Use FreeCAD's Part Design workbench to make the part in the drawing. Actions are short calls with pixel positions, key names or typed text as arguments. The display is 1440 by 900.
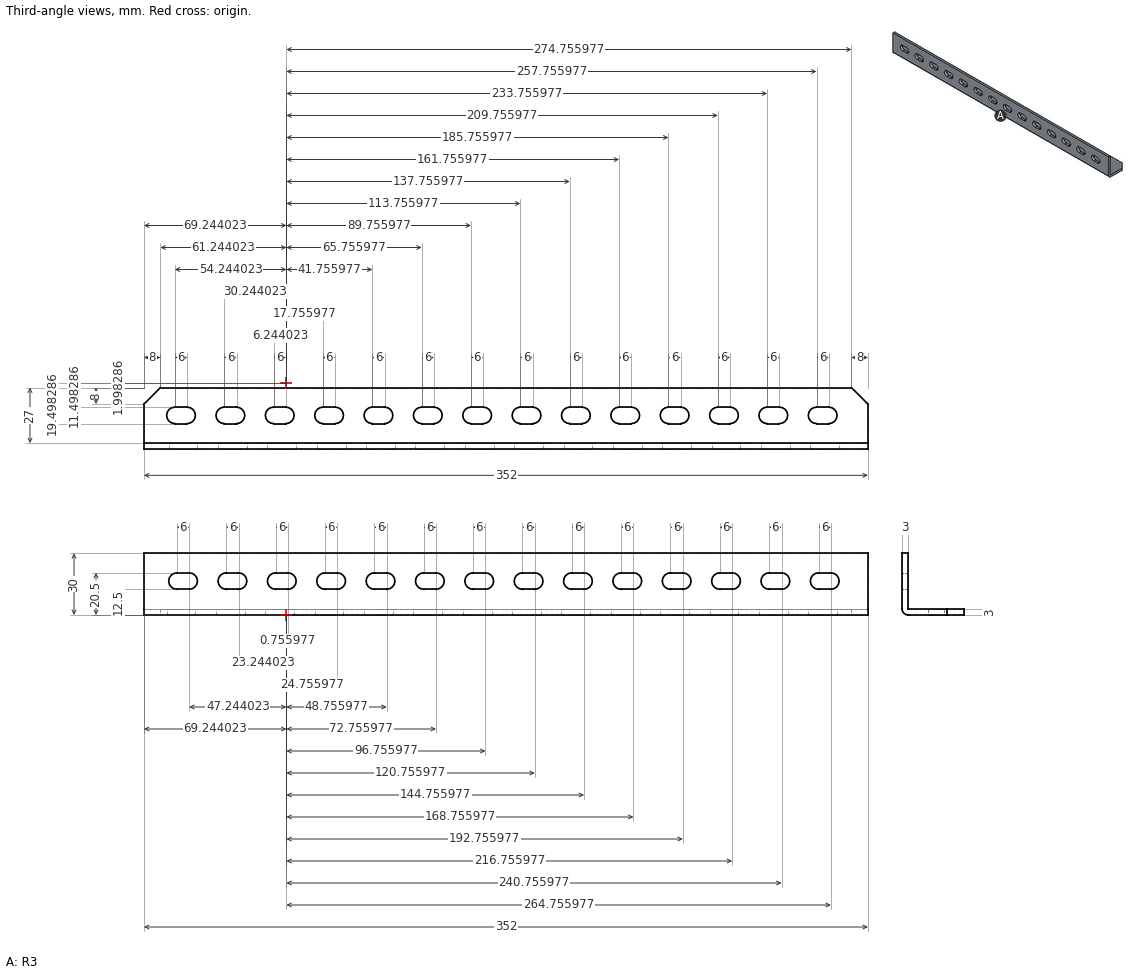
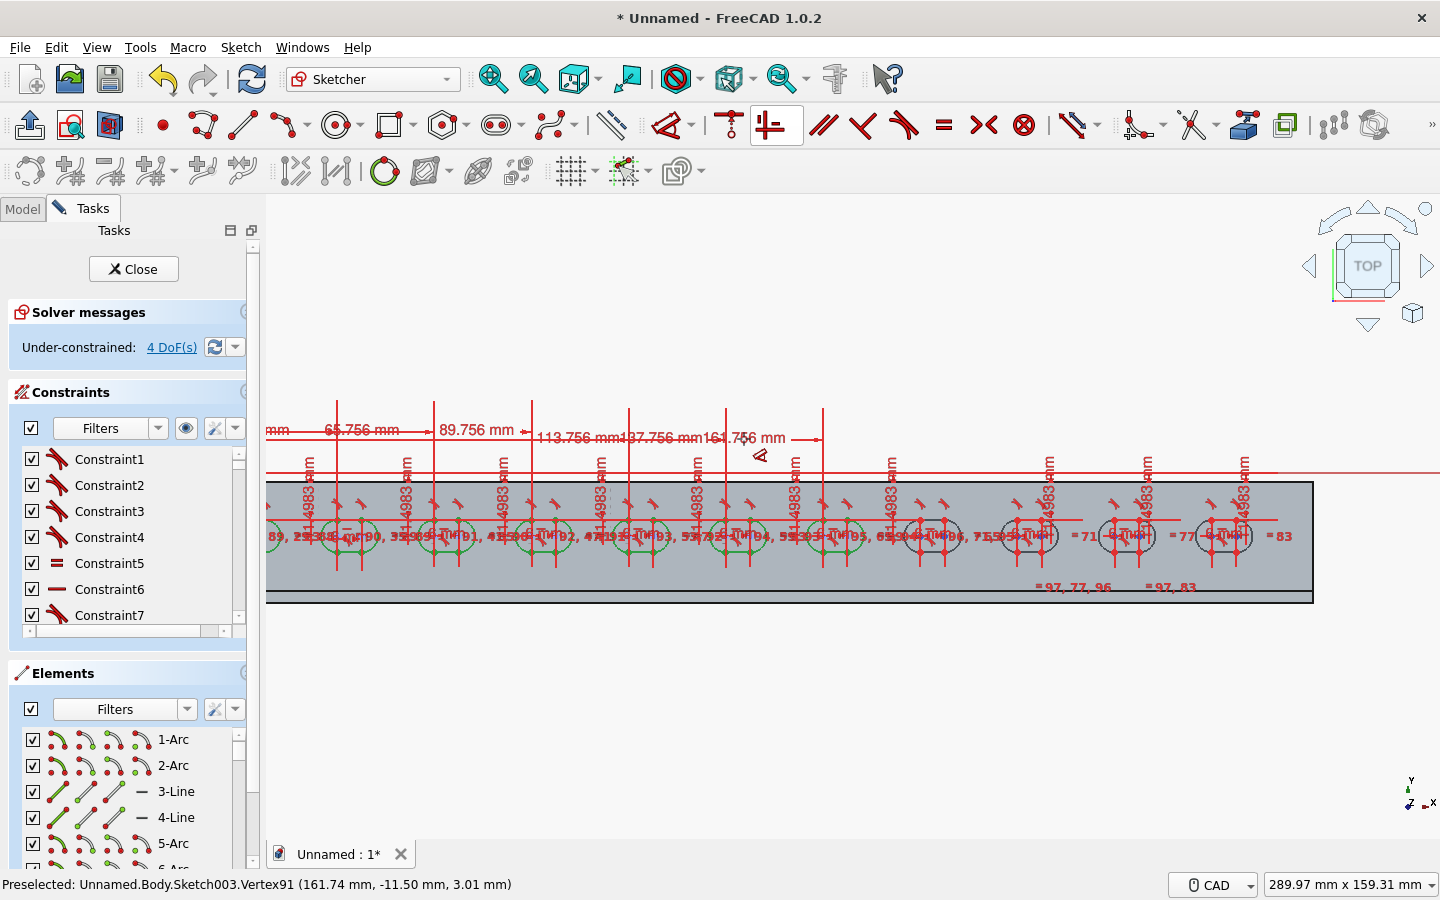
click(920, 520)
click(826, 439)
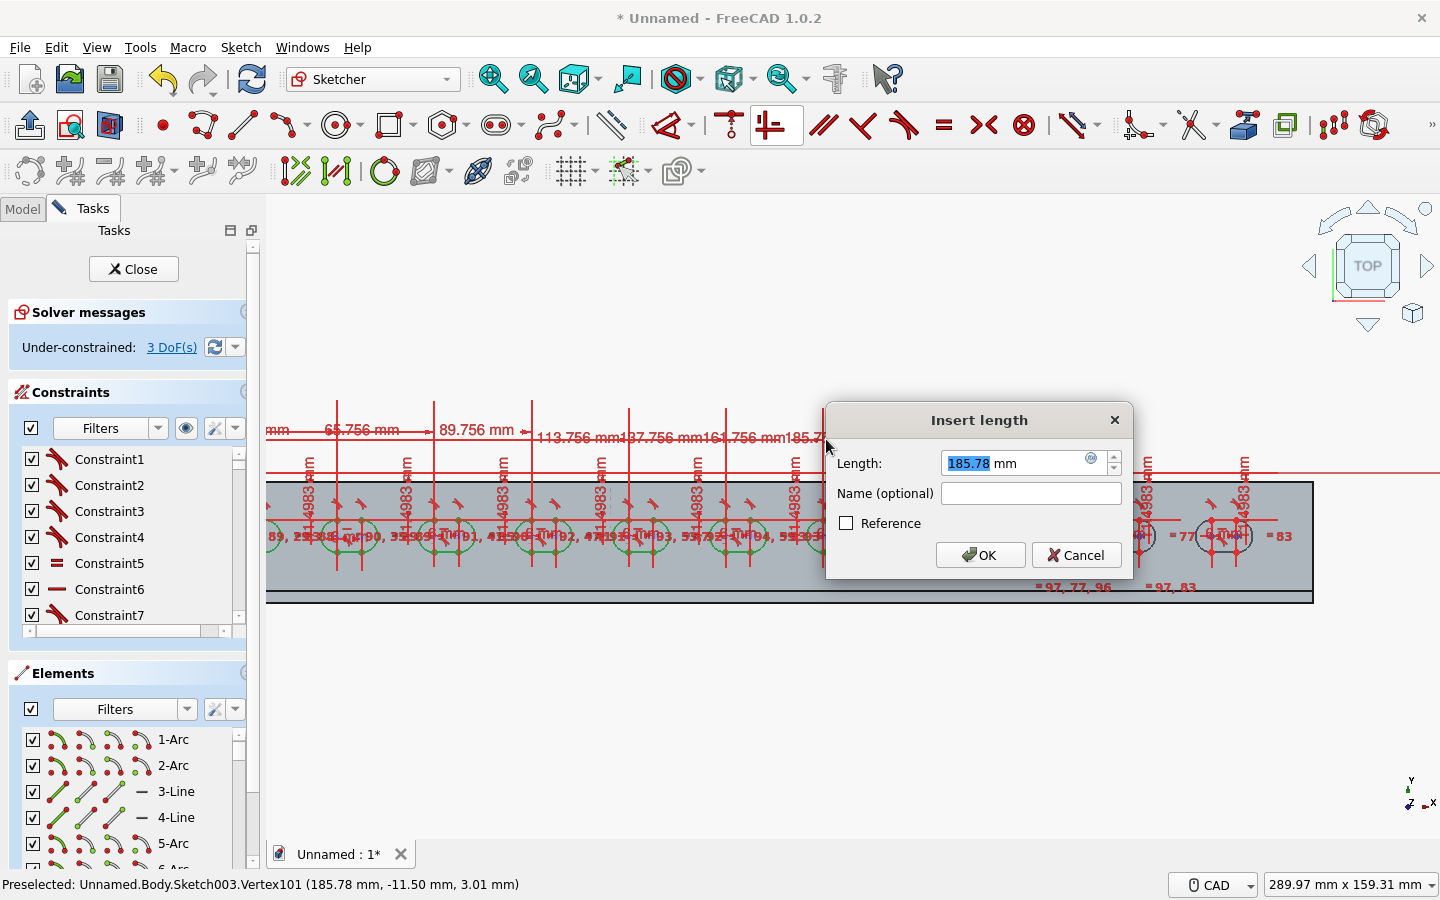
text(185.755977)
key(Return)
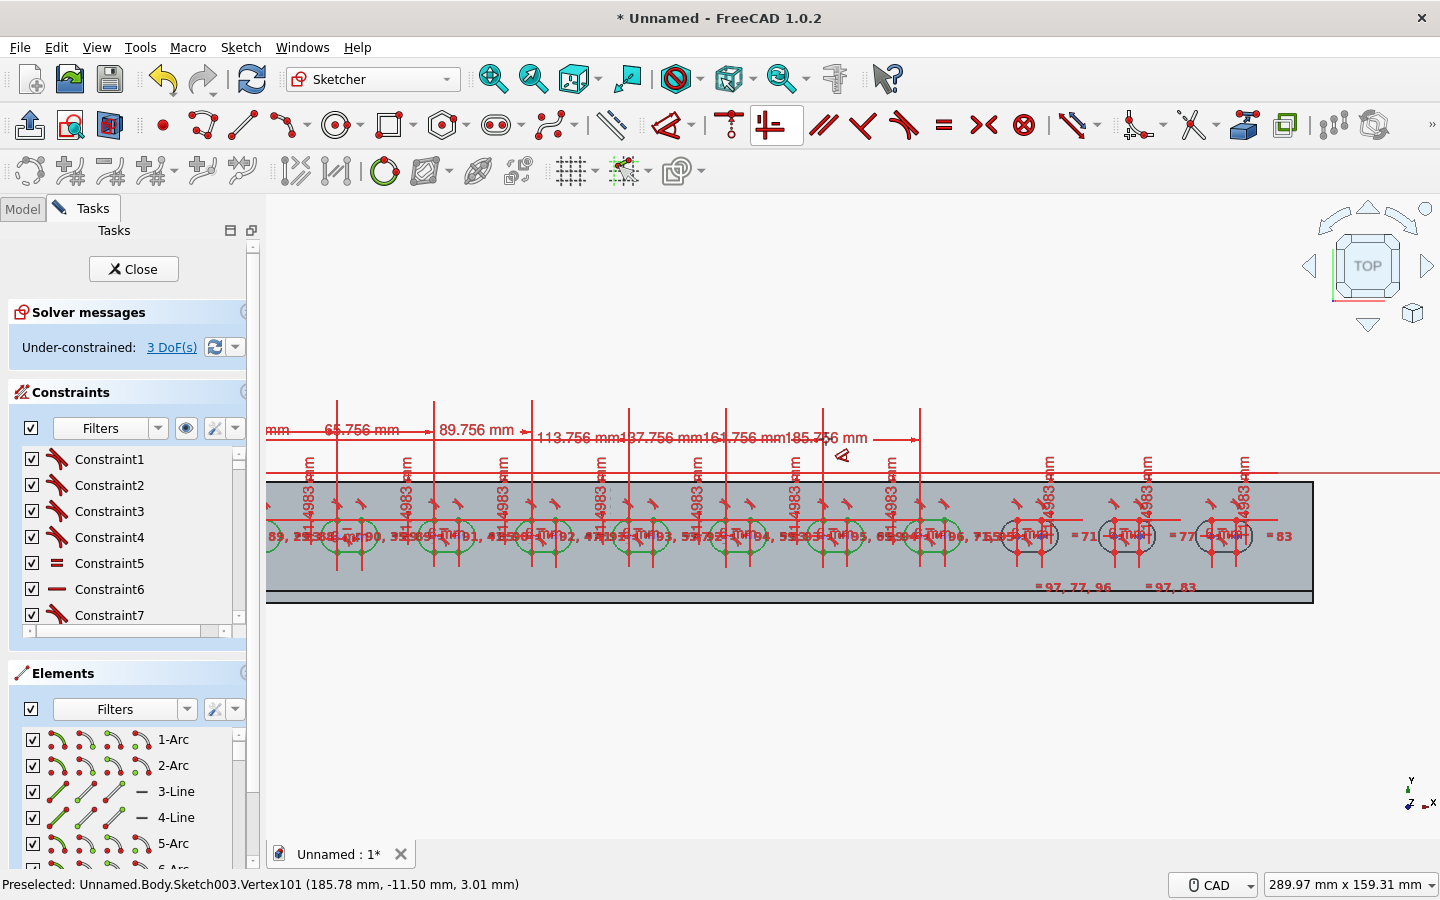
click(1017, 520)
click(909, 439)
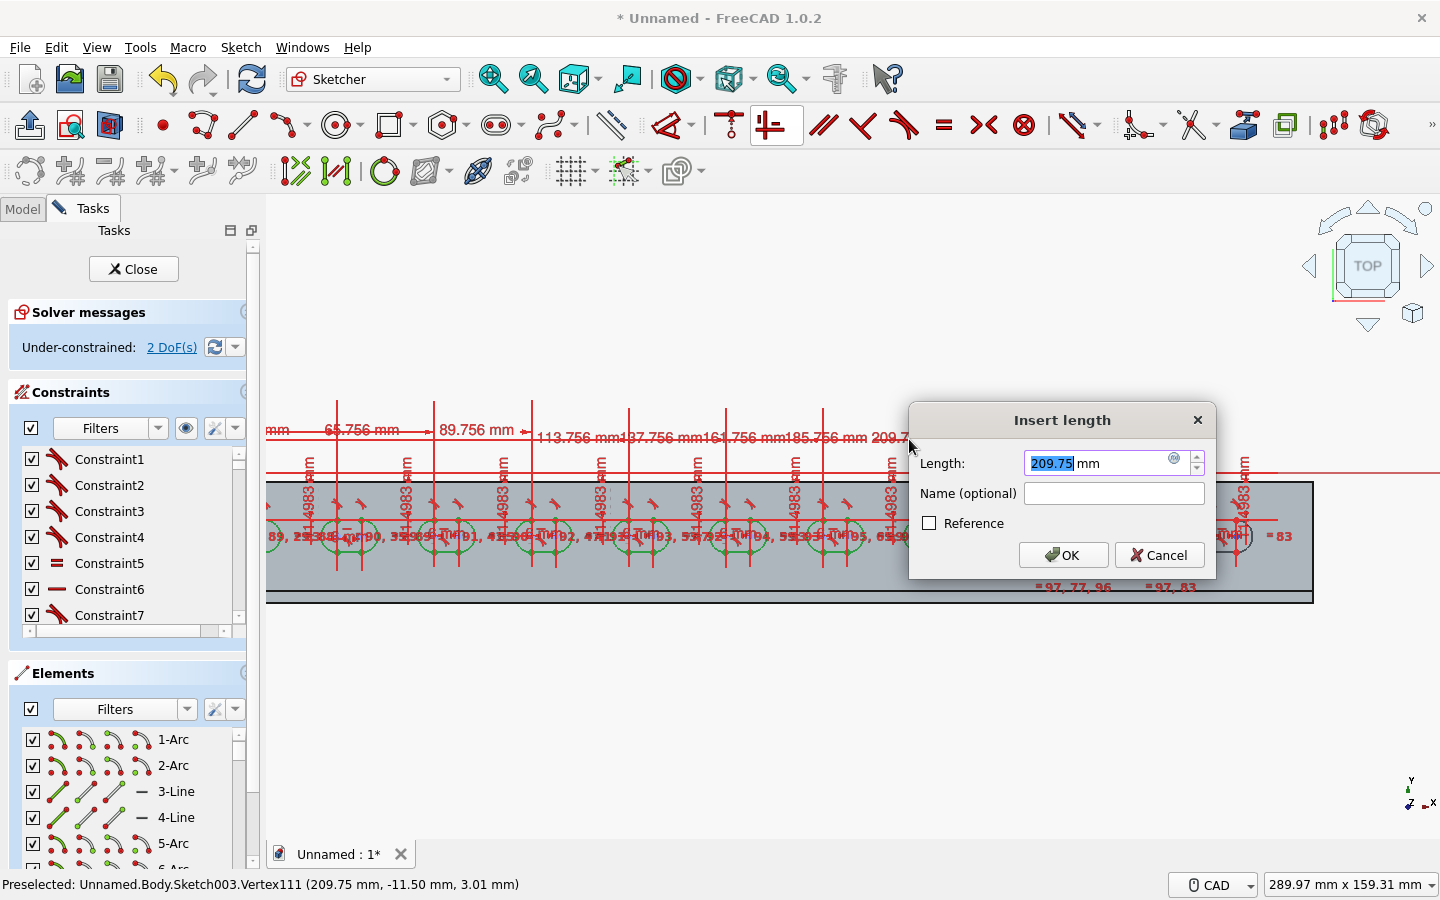
text(209.755977)
key(Return)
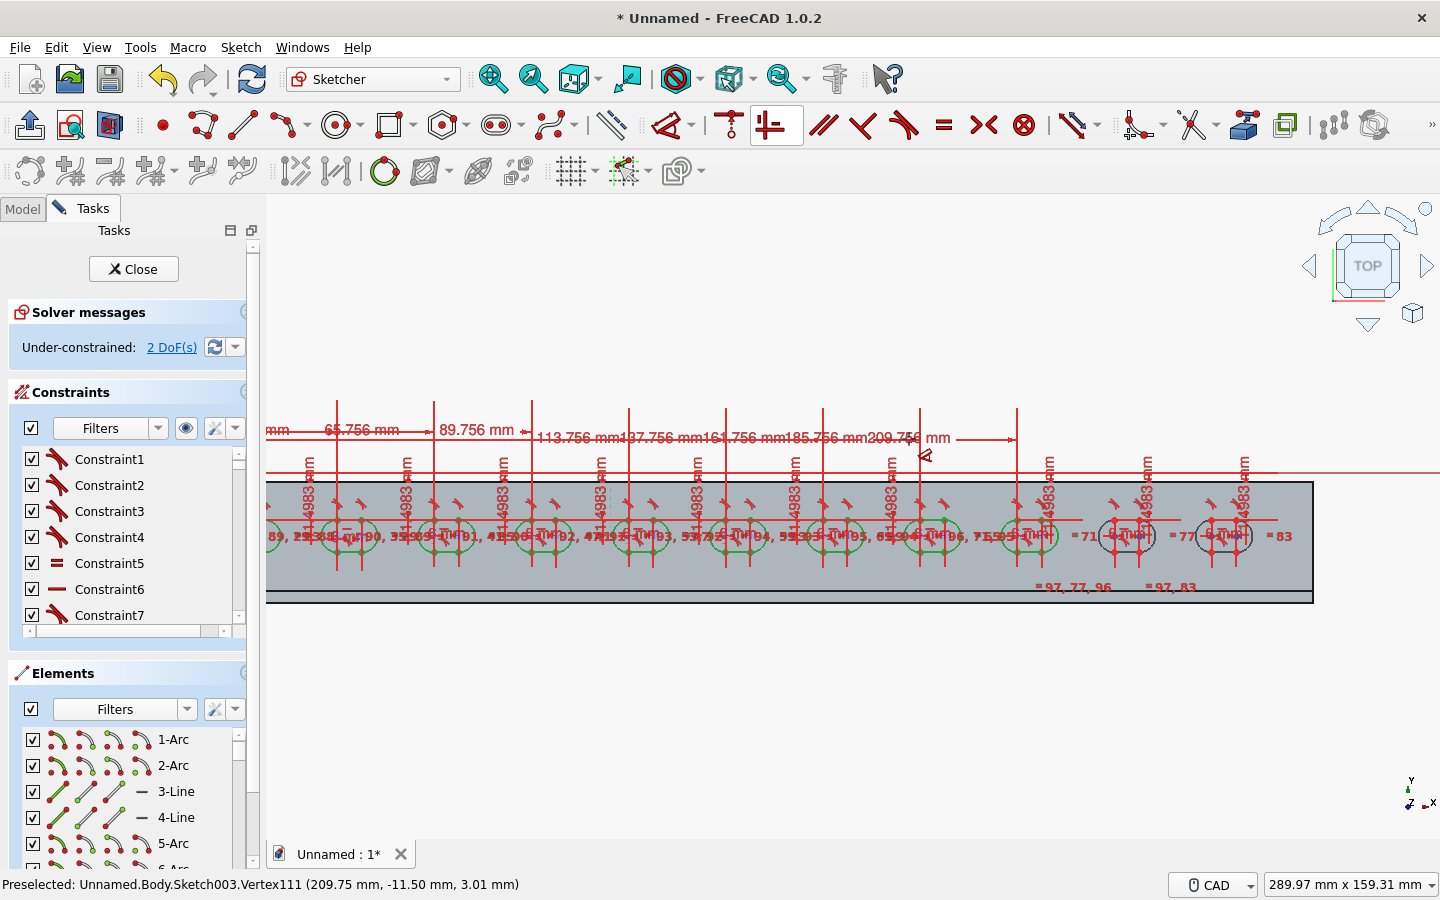
click(1115, 520)
click(992, 439)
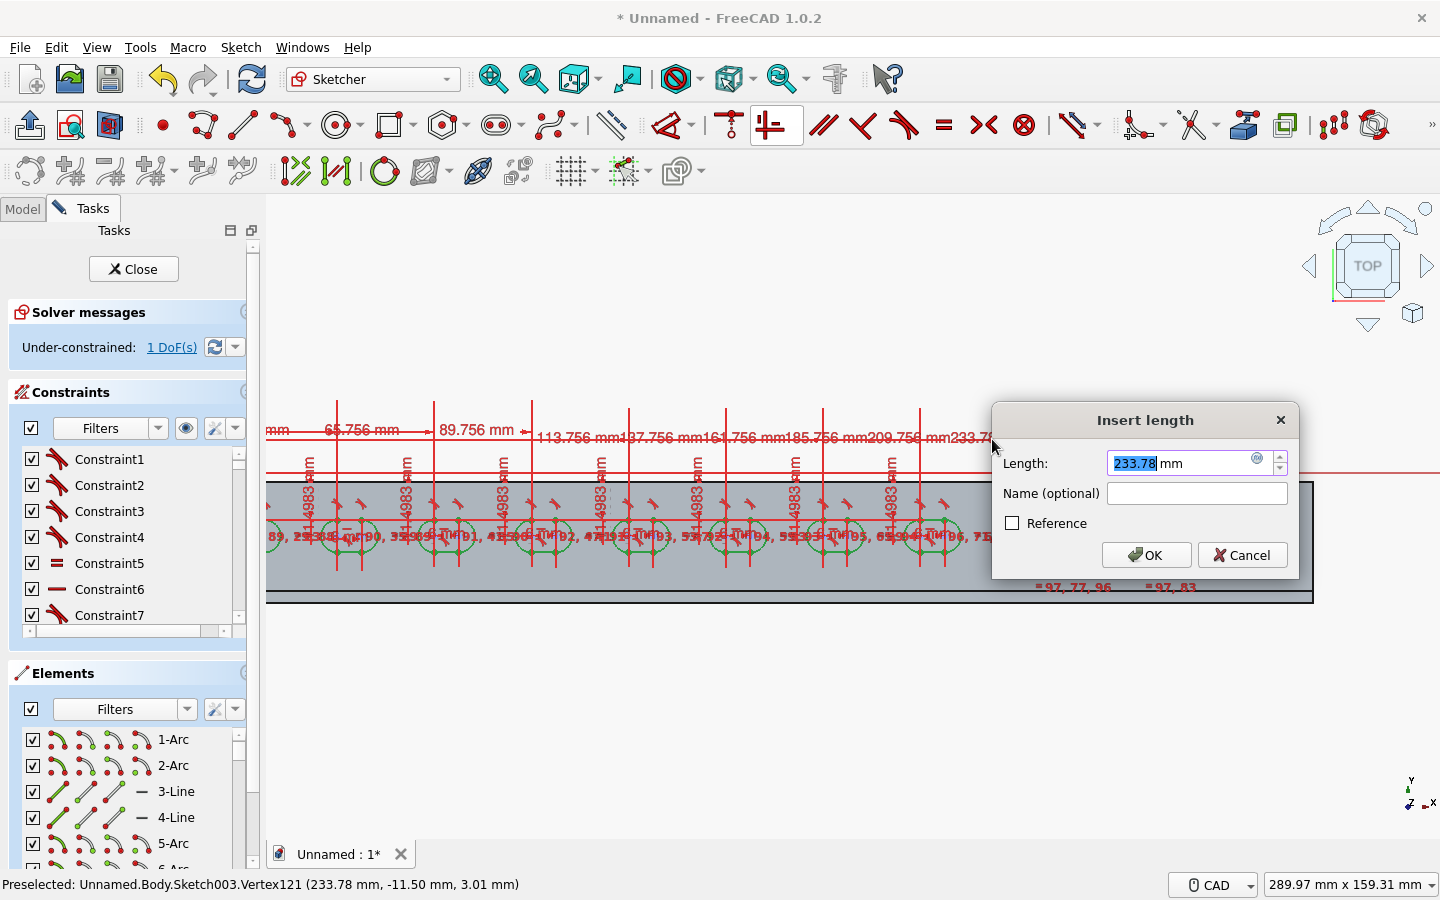
text(233.755977)
key(Return)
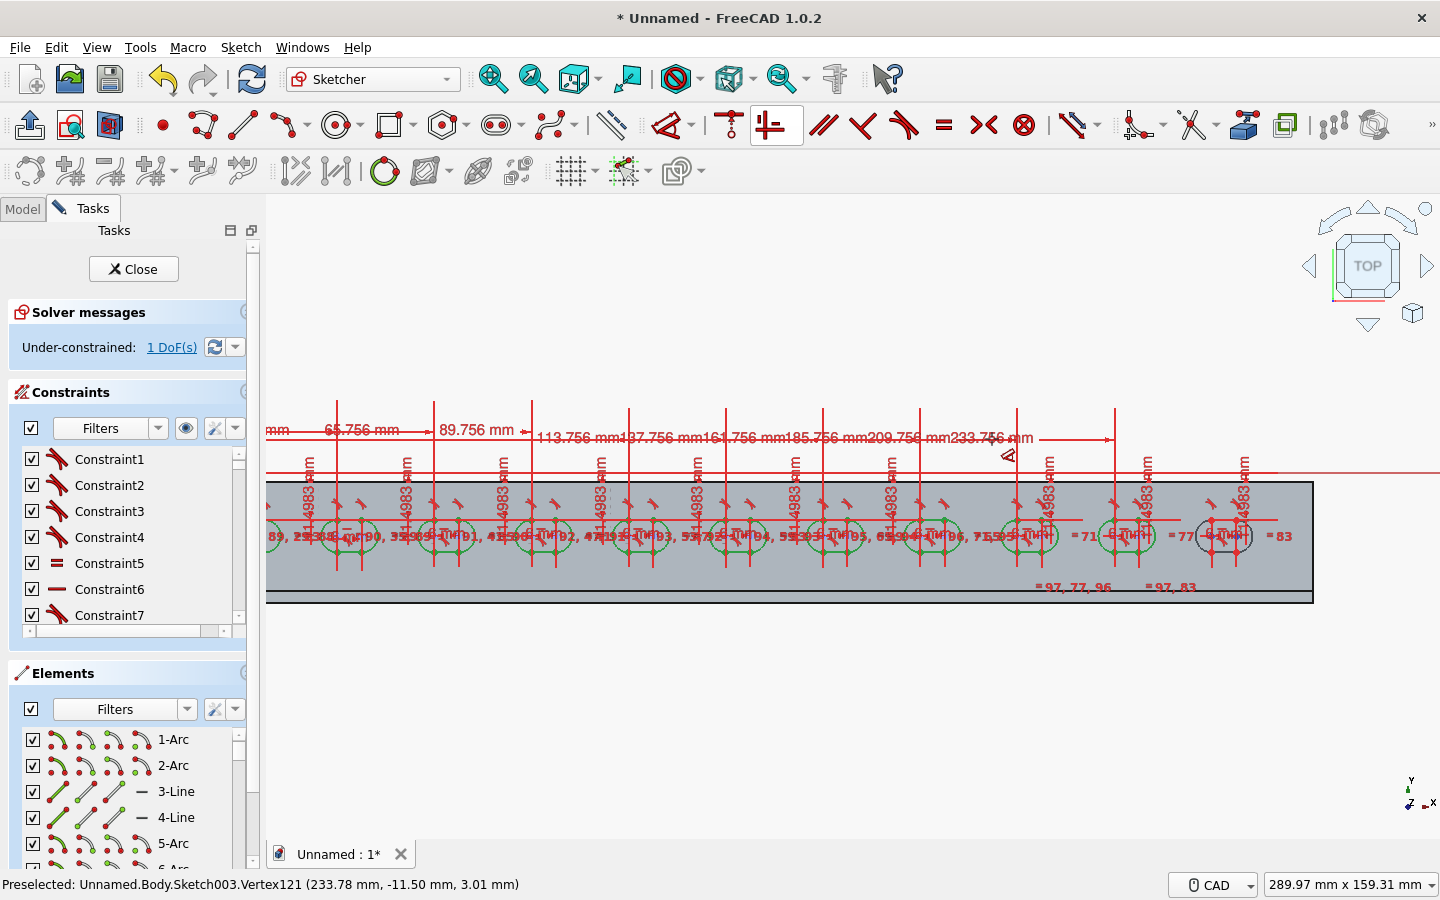
click(1212, 520)
click(1074, 439)